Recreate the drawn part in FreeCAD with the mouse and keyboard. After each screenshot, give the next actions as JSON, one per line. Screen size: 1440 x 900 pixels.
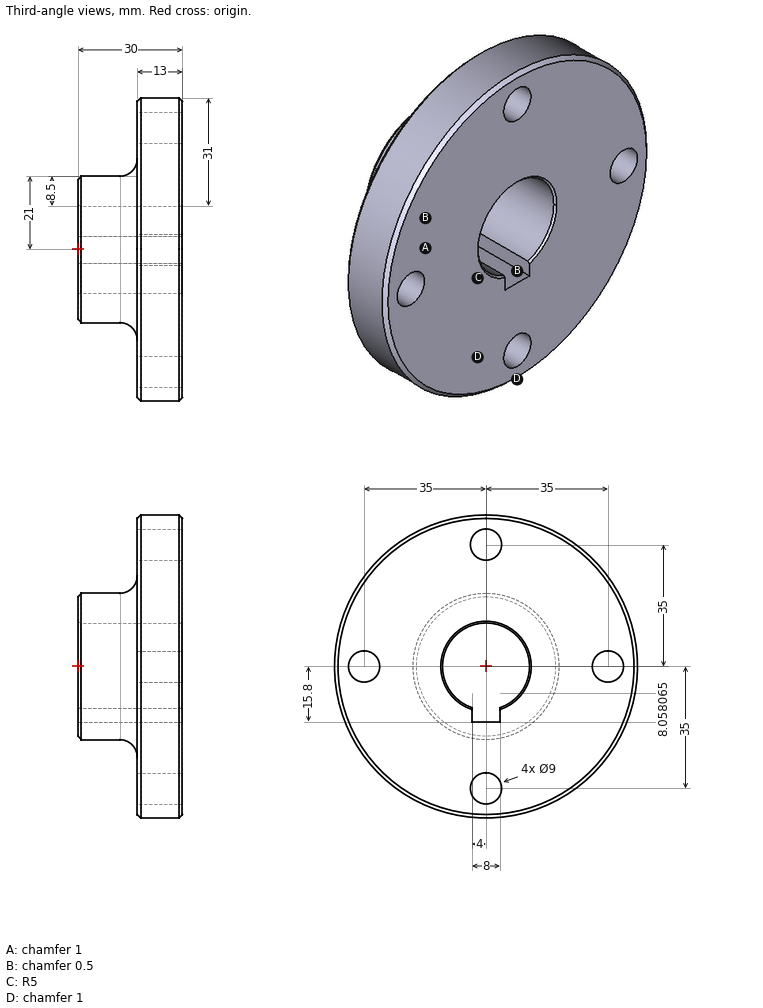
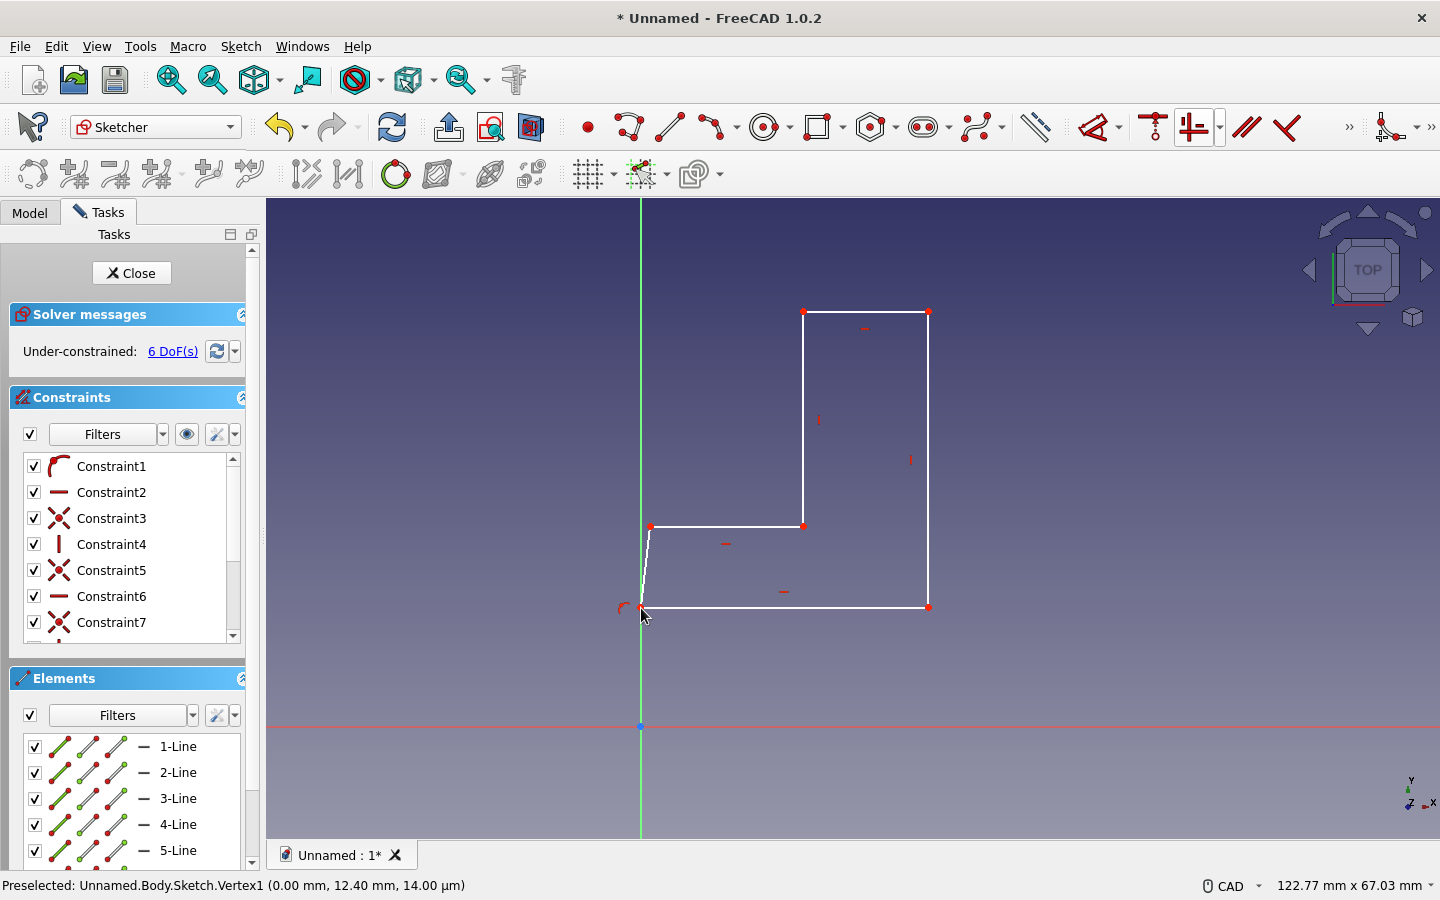
{"action": "left_click", "coordinate": [644, 584]}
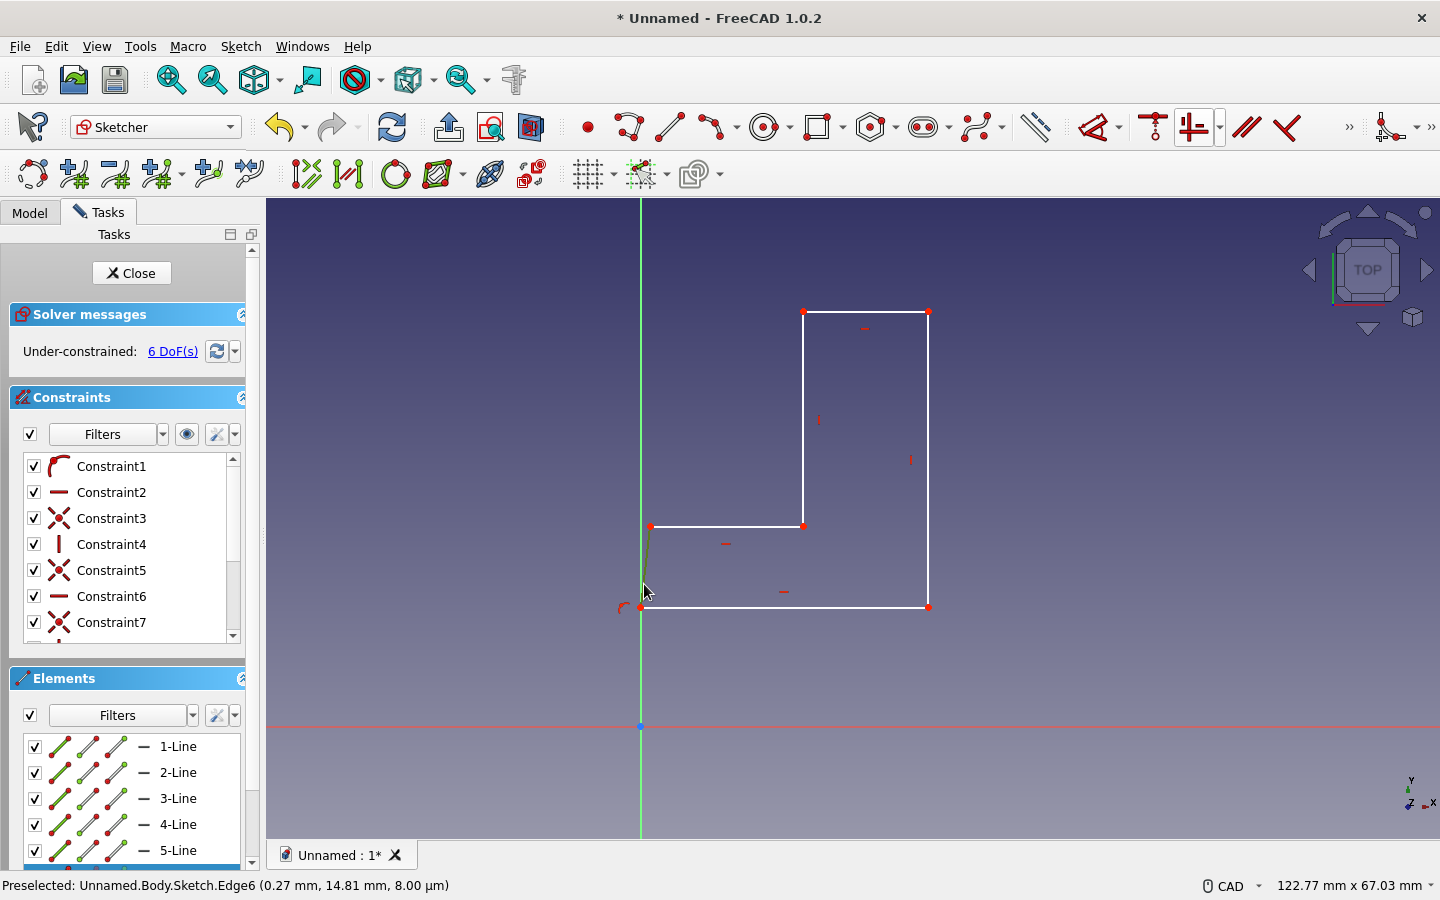
{"action": "key", "text": "v"}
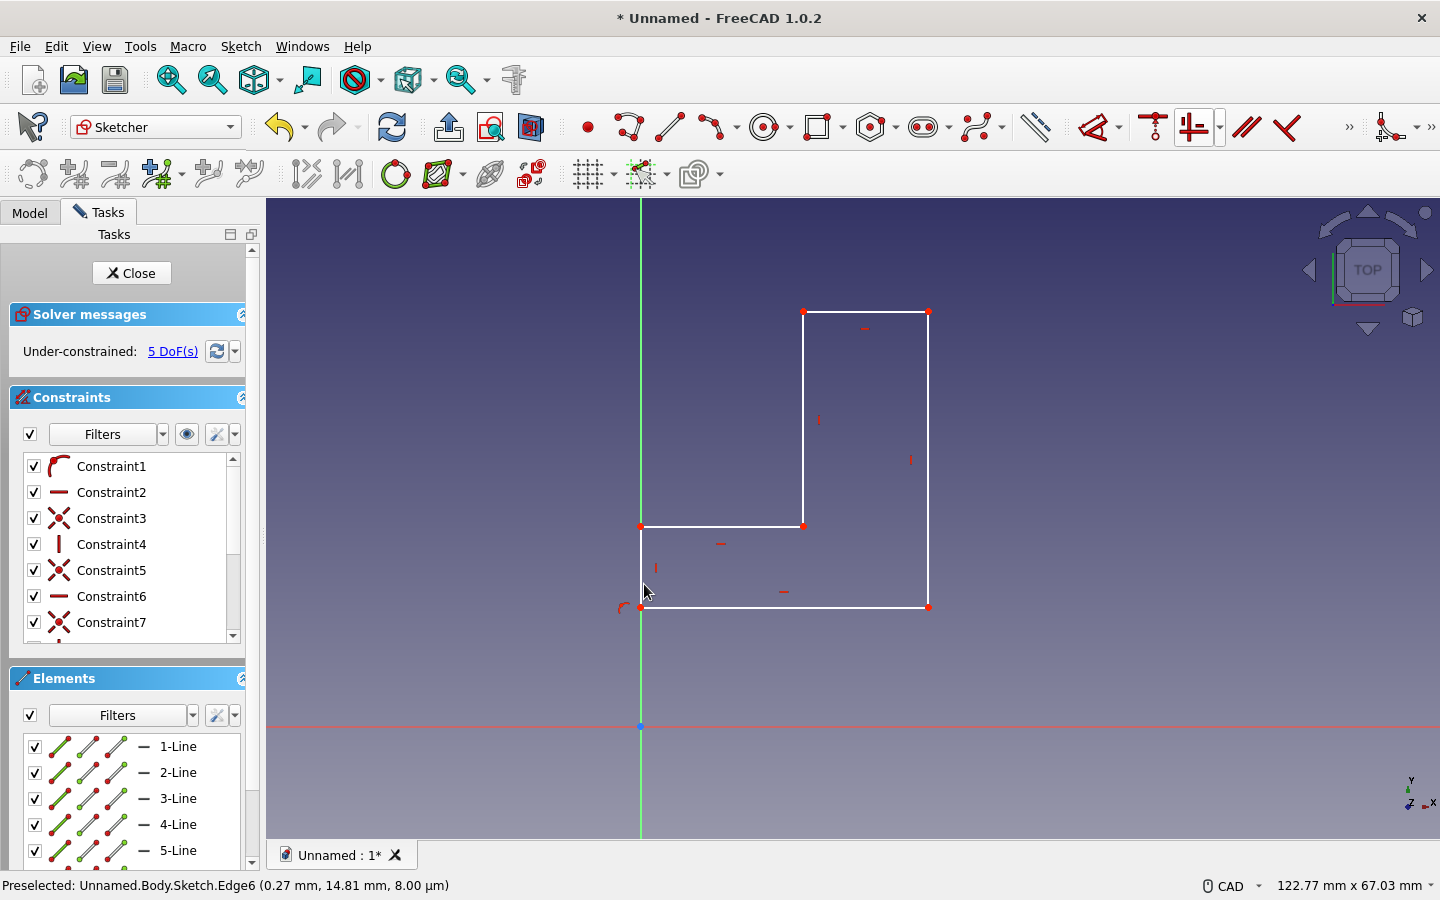
{"action": "left_click", "coordinate": [1092, 128]}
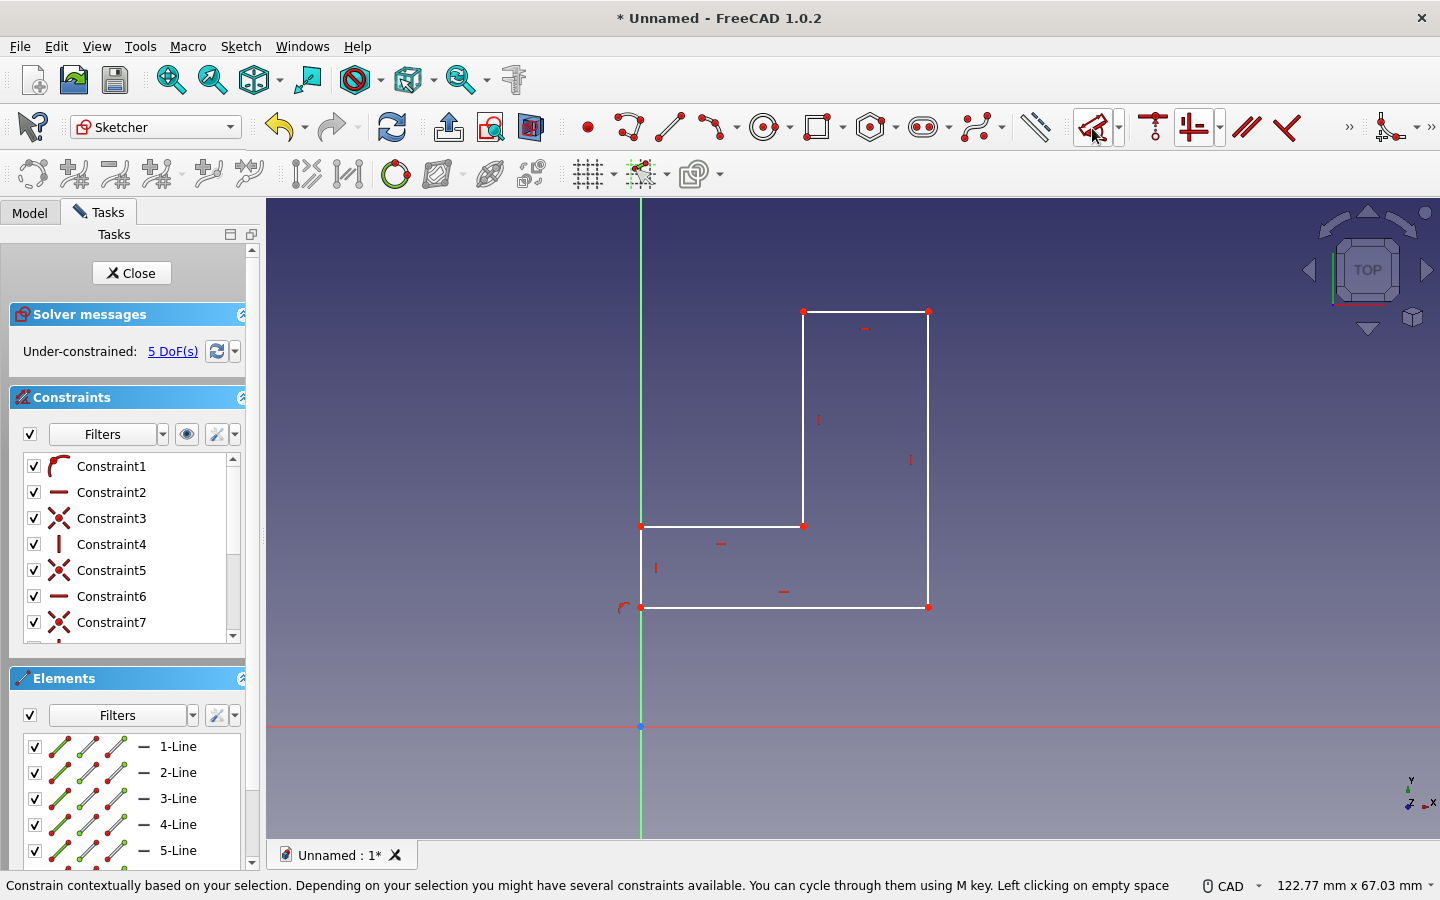
{"action": "left_click", "coordinate": [727, 608]}
{"action": "left_click", "coordinate": [784, 642]}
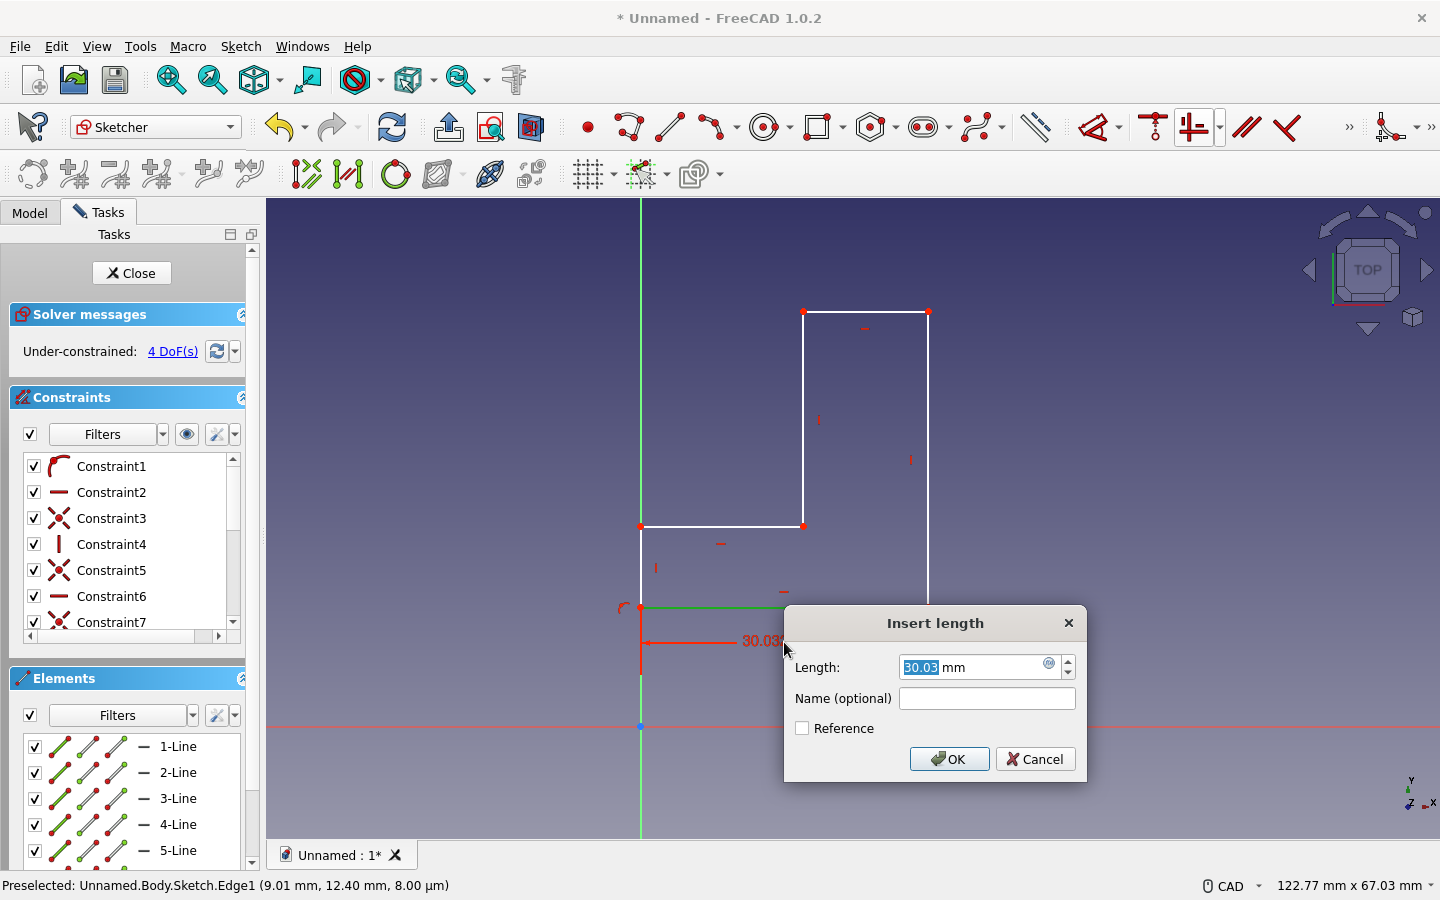
{"action": "type", "text": "30"}
{"action": "key", "text": "Return"}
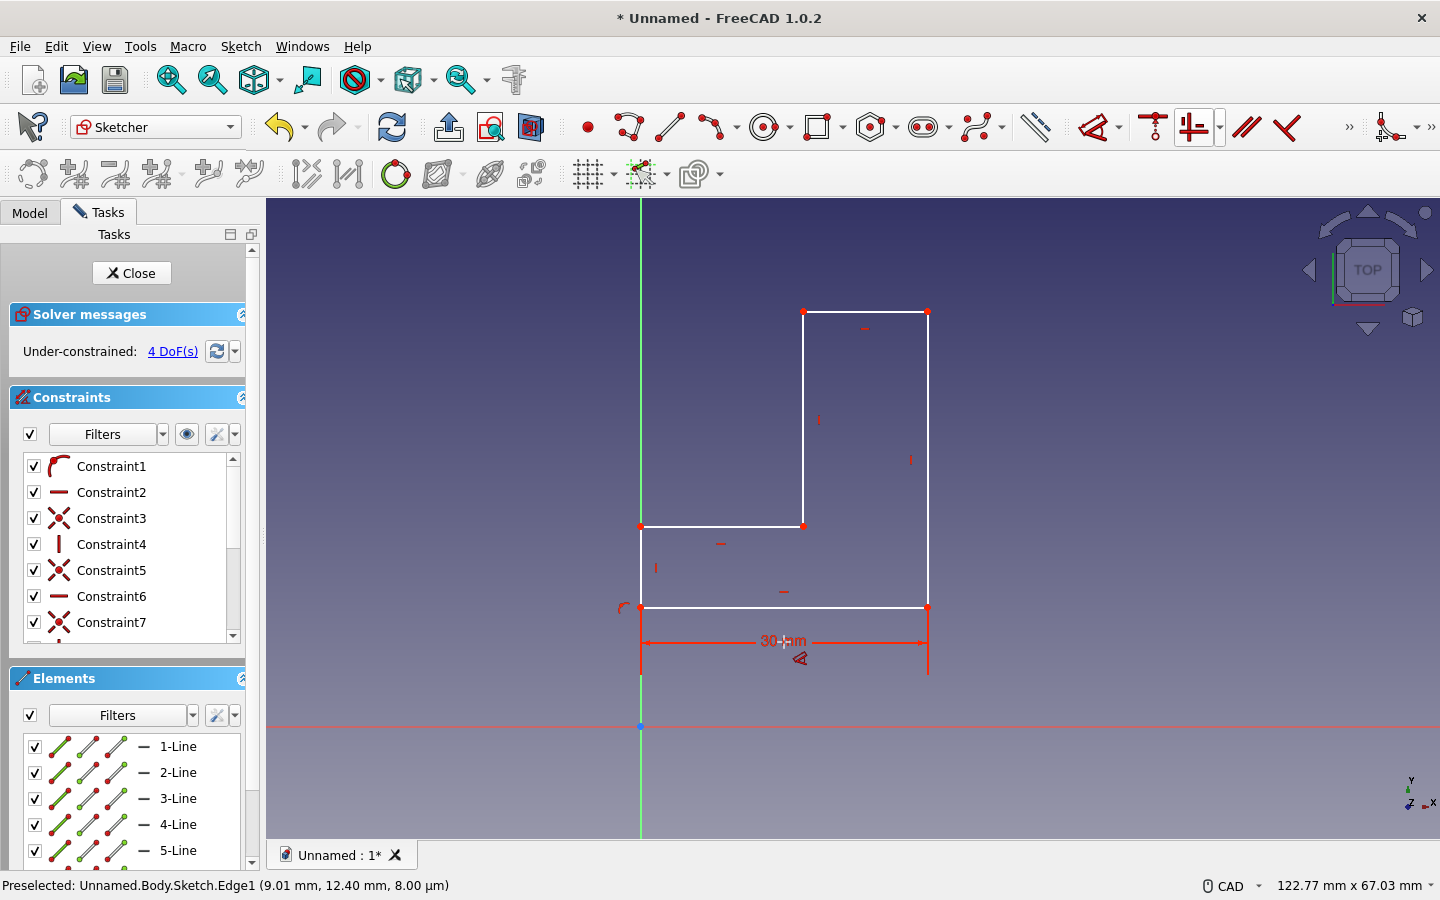
{"action": "left_click", "coordinate": [928, 519]}
{"action": "left_click", "coordinate": [962, 460]}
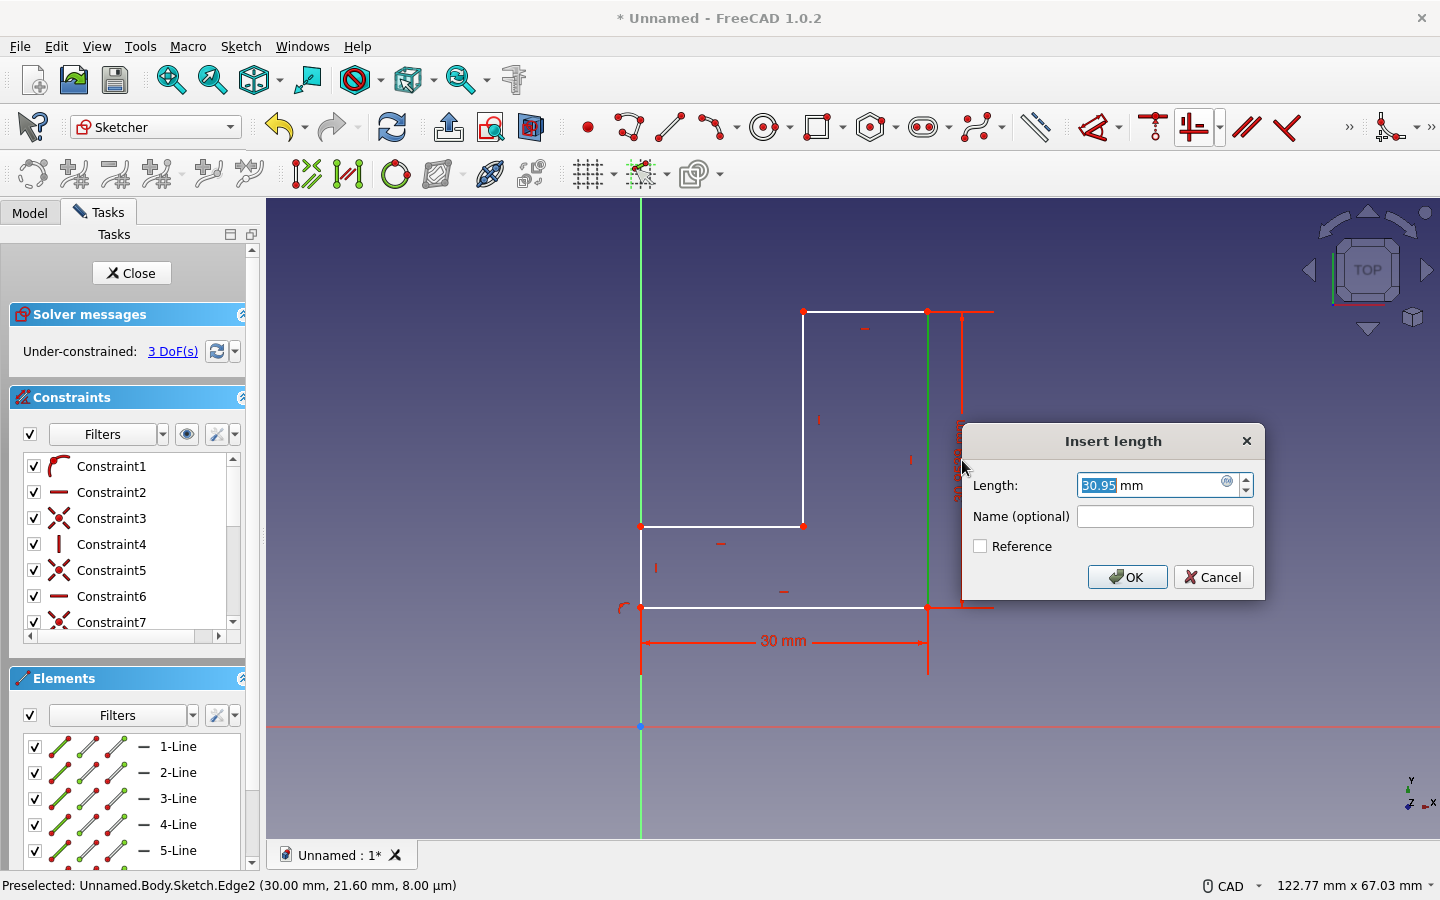
{"action": "type", "text": "31"}
{"action": "key", "text": "Return"}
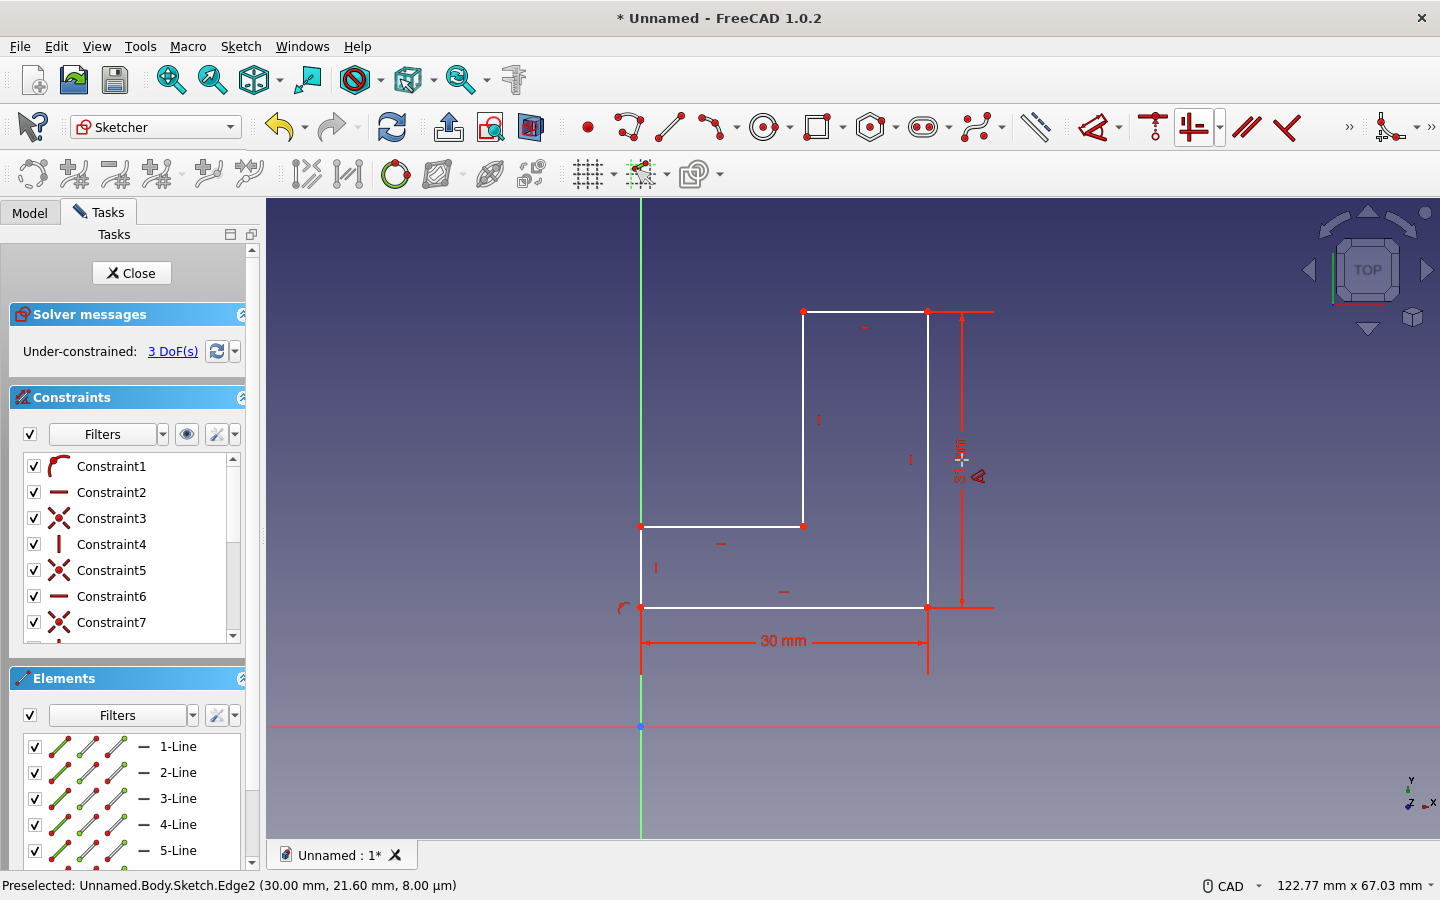
{"action": "left_click", "coordinate": [890, 312]}
{"action": "left_click", "coordinate": [865, 278]}